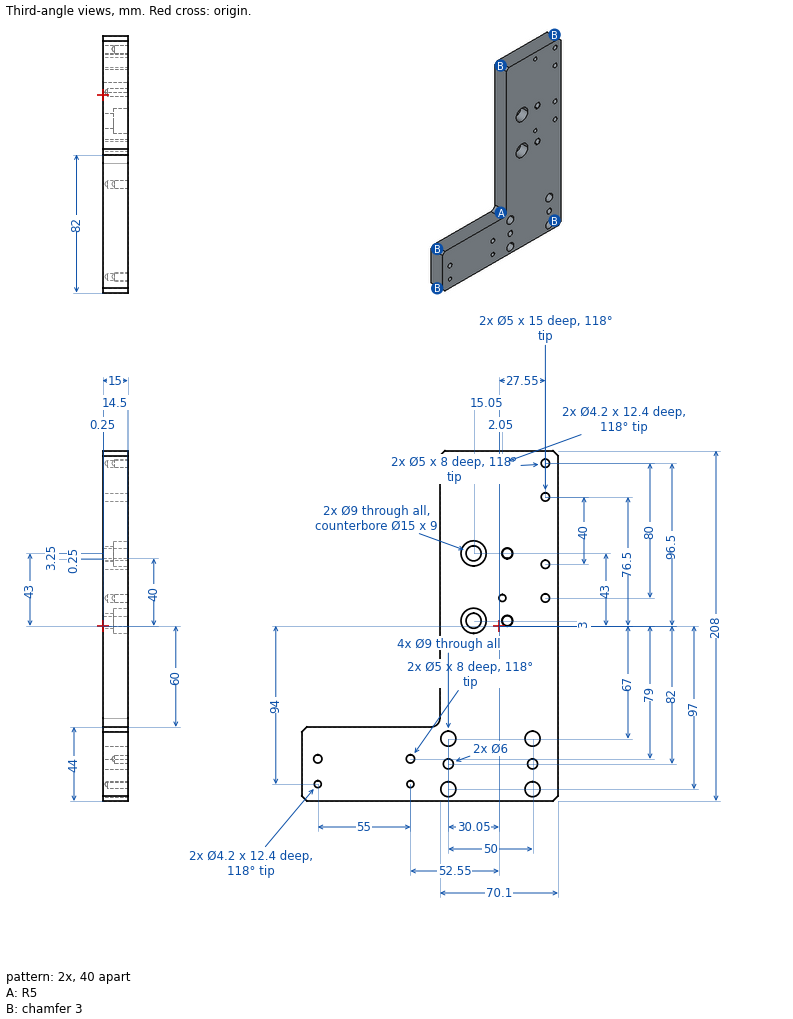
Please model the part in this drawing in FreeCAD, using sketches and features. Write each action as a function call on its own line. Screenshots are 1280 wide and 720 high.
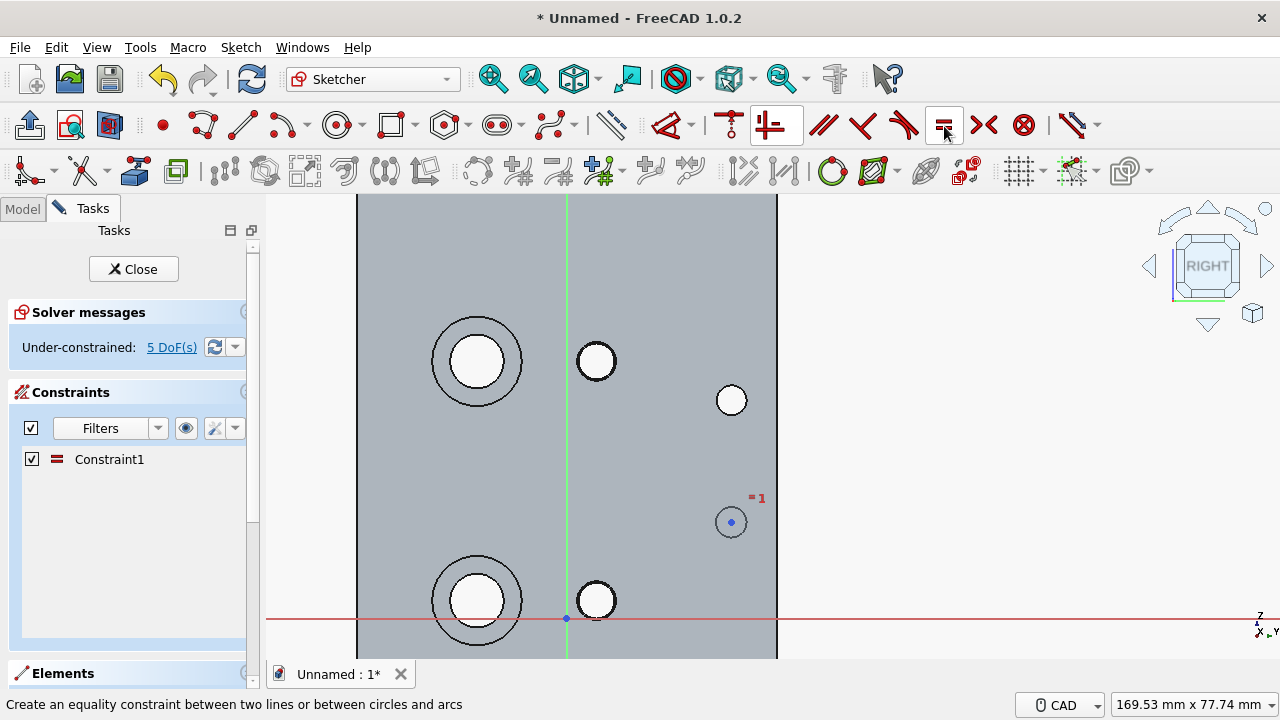
scroll(743, 511, down, 4)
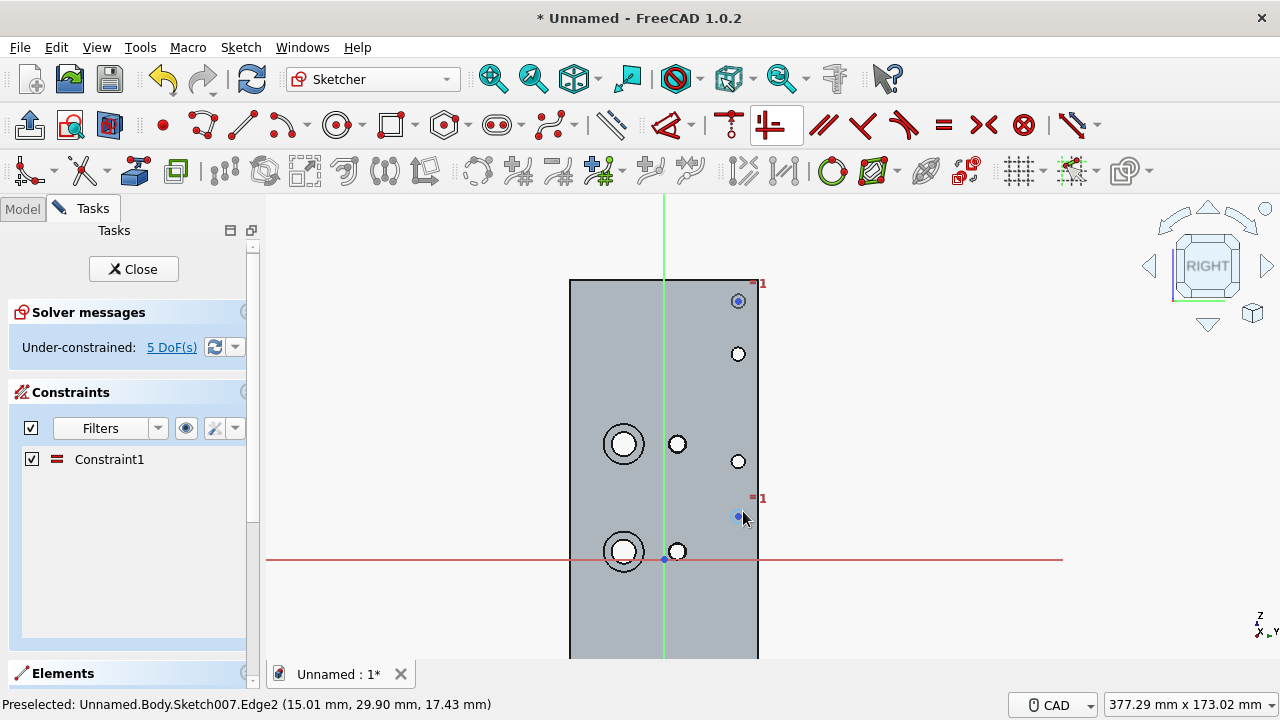
click(738, 301)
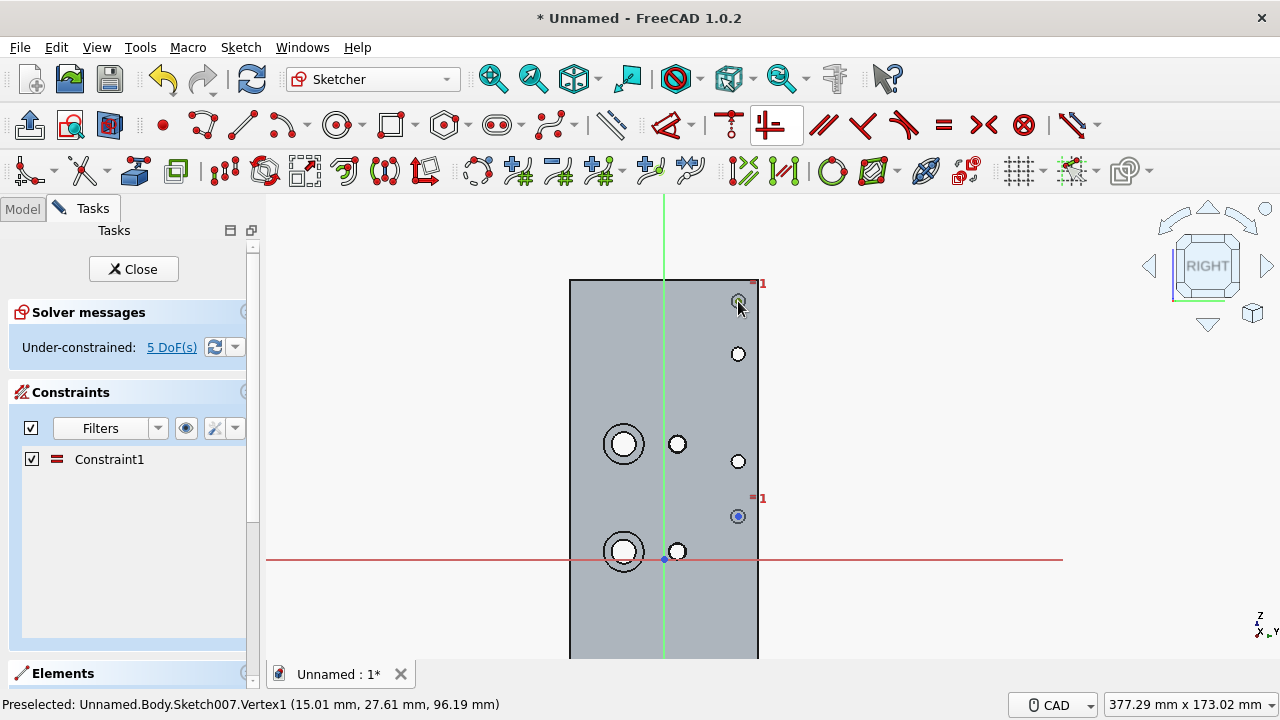
click(738, 516)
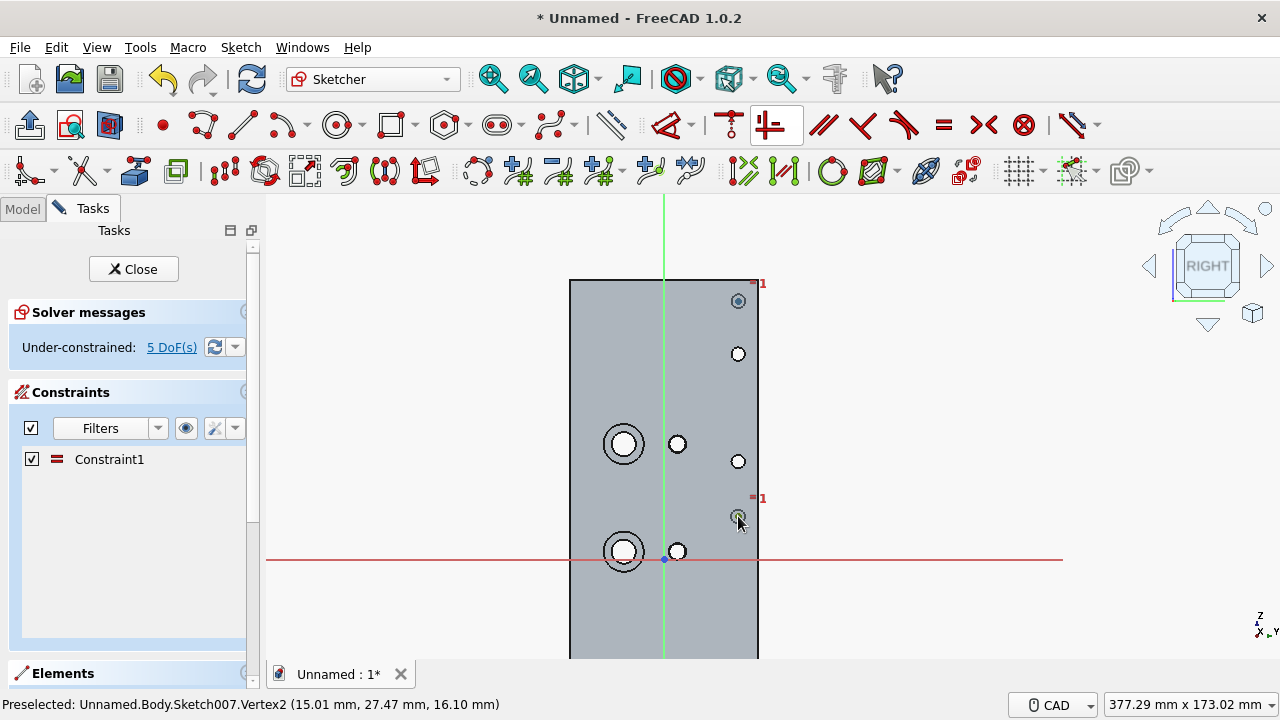
click(798, 126)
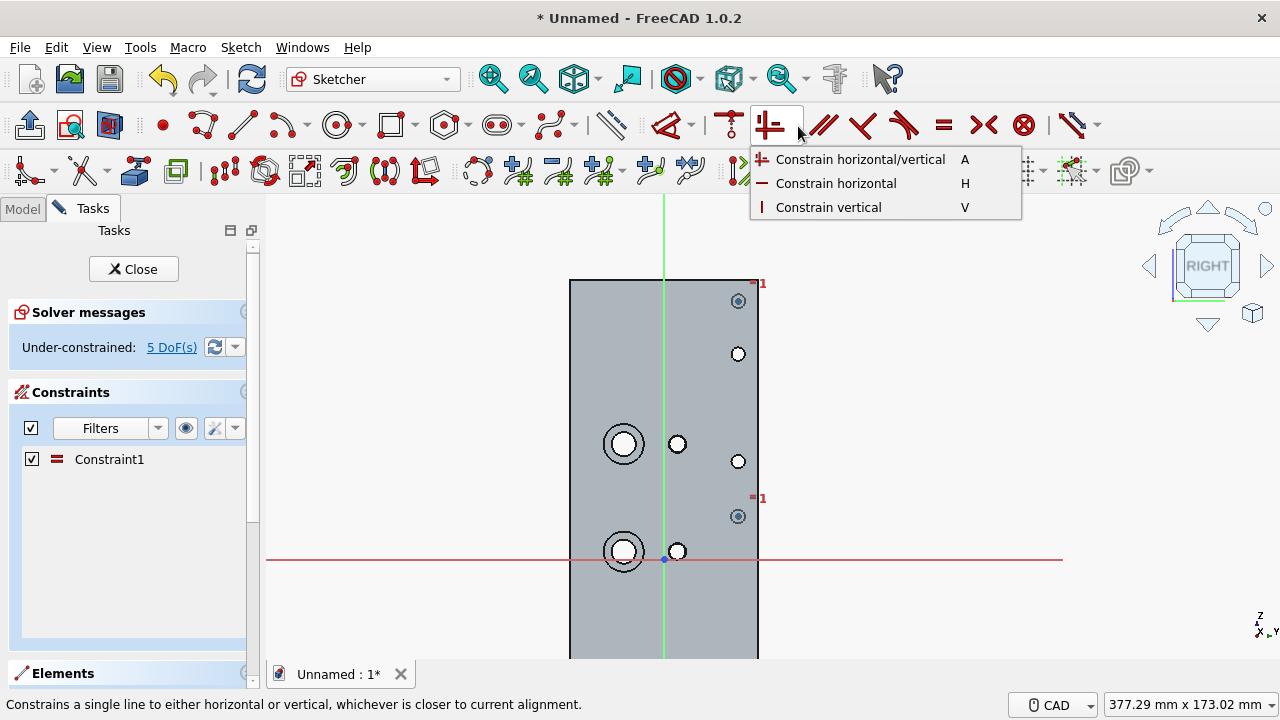
click(886, 207)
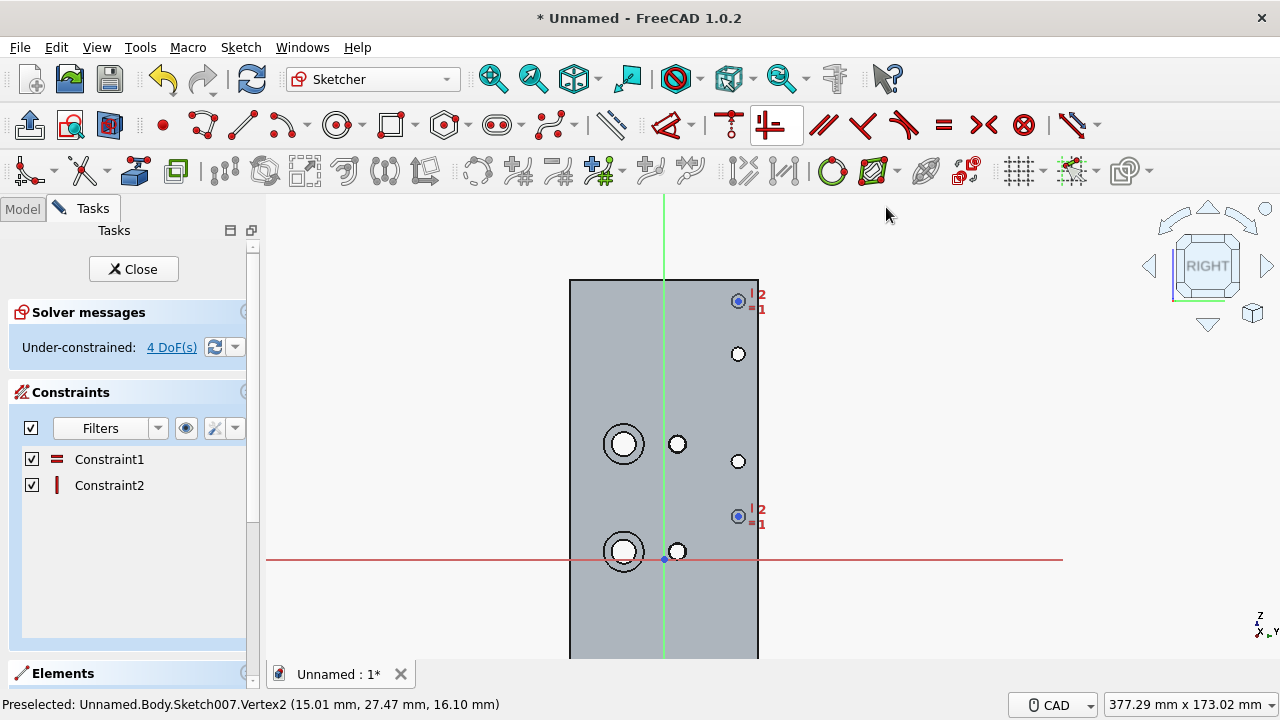
click(666, 126)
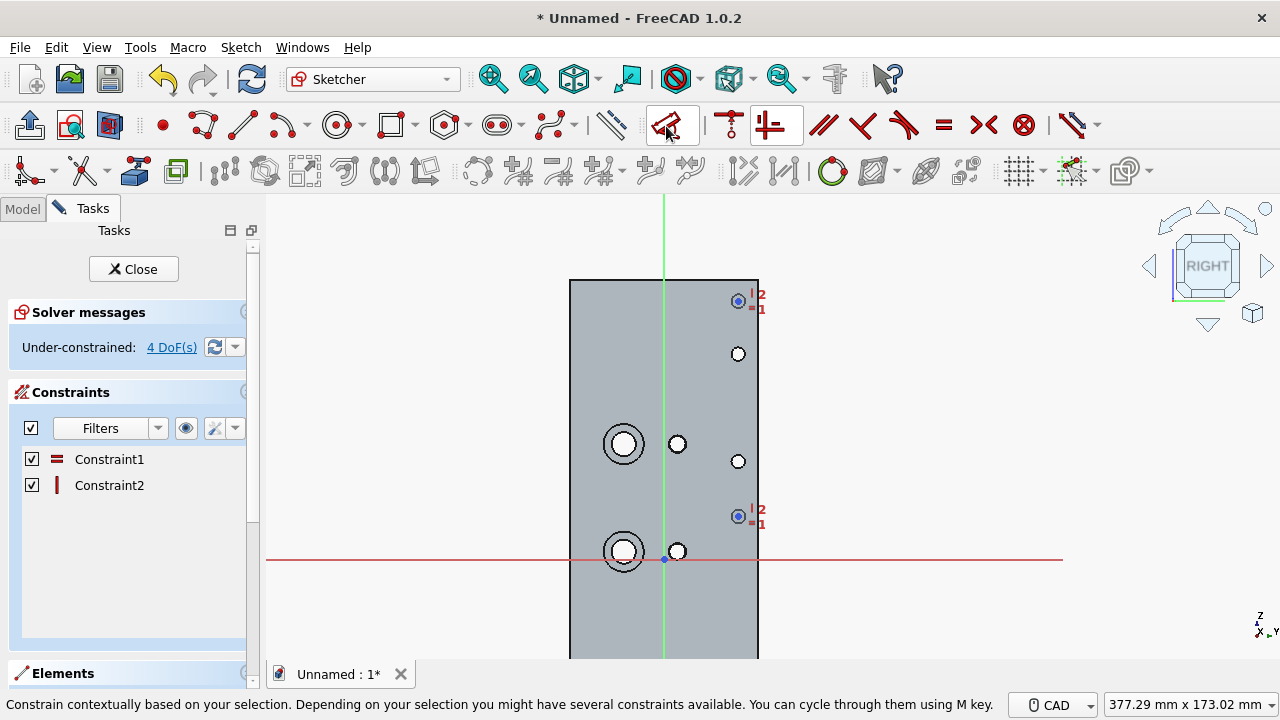
scroll(745, 301, up, 6)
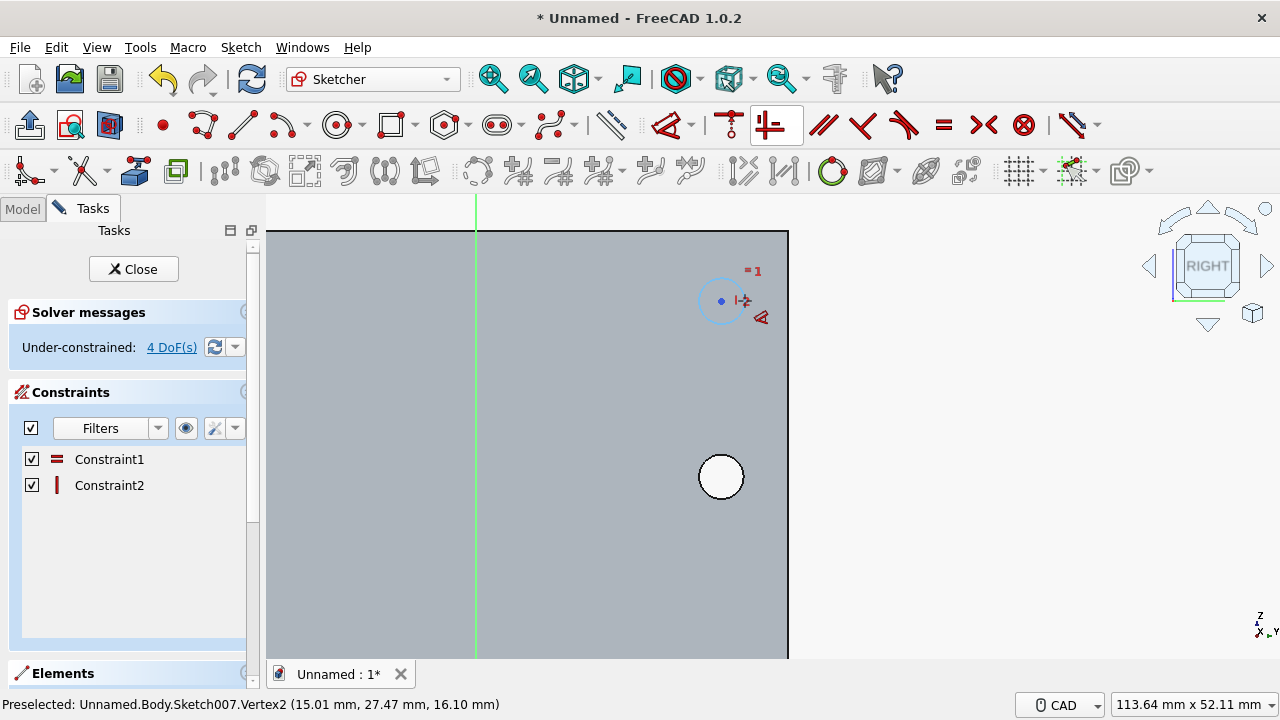
click(745, 302)
click(777, 303)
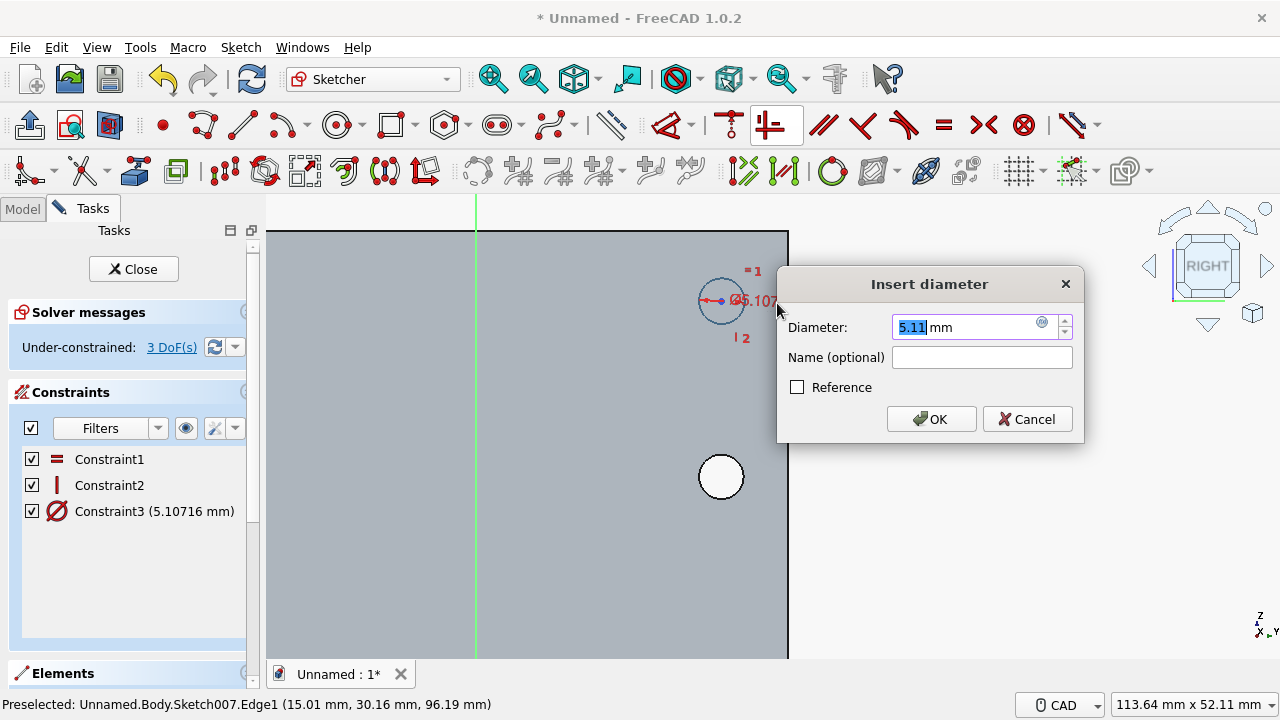
text(5)
key(Return)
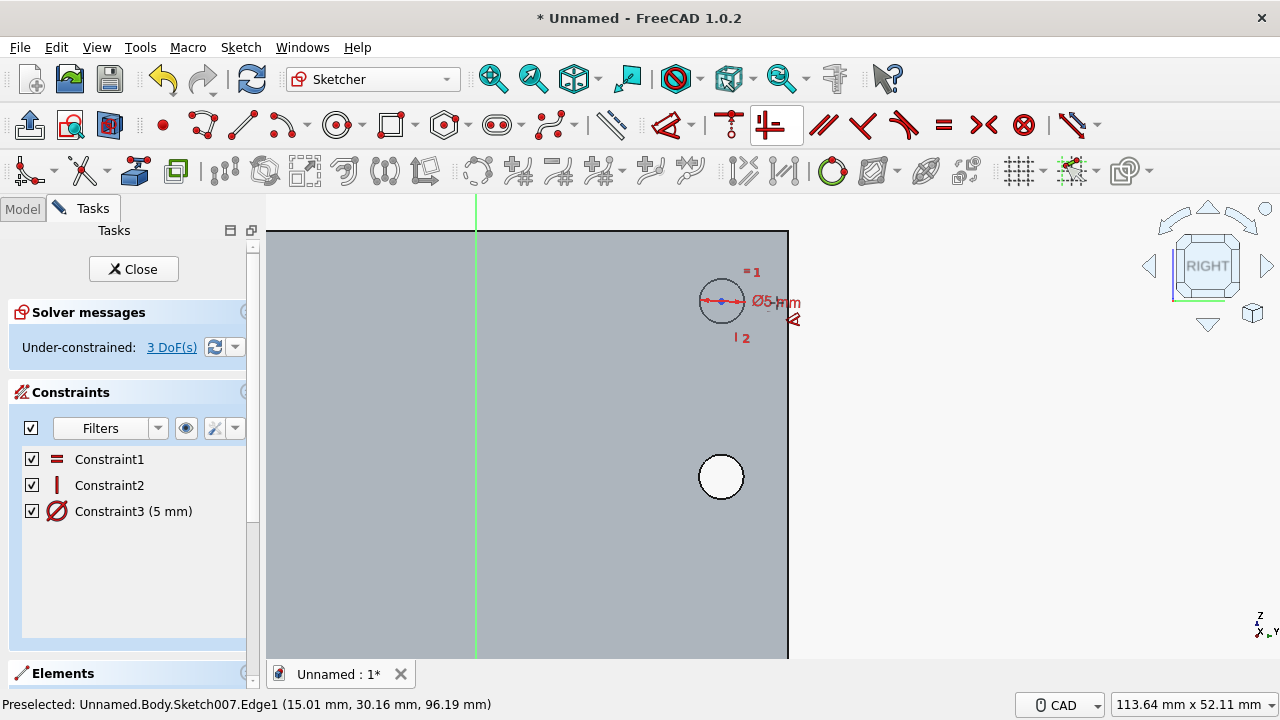
click(722, 301)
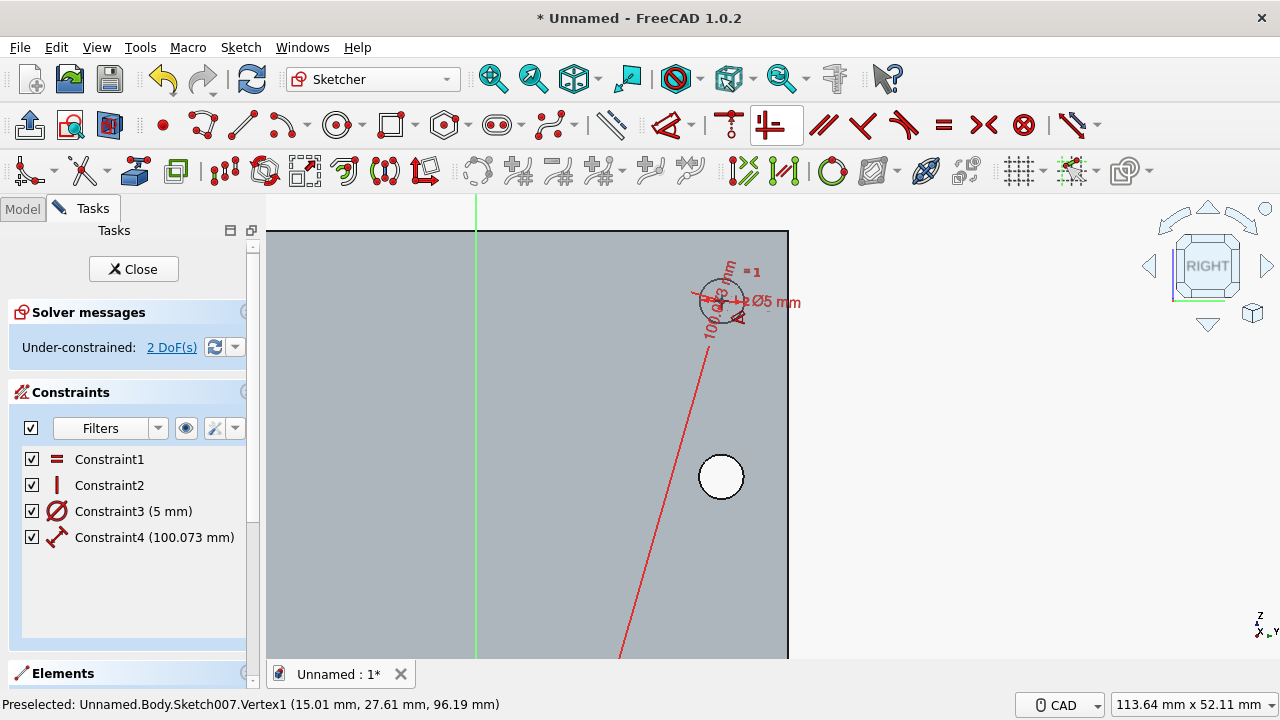
scroll(745, 301, down, 6)